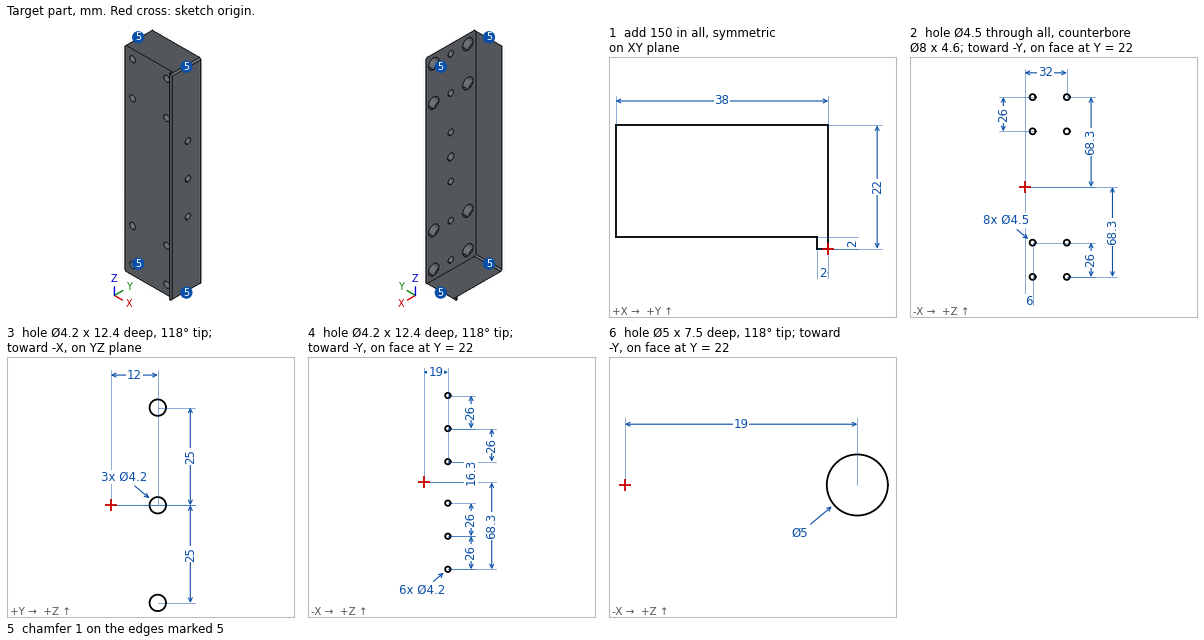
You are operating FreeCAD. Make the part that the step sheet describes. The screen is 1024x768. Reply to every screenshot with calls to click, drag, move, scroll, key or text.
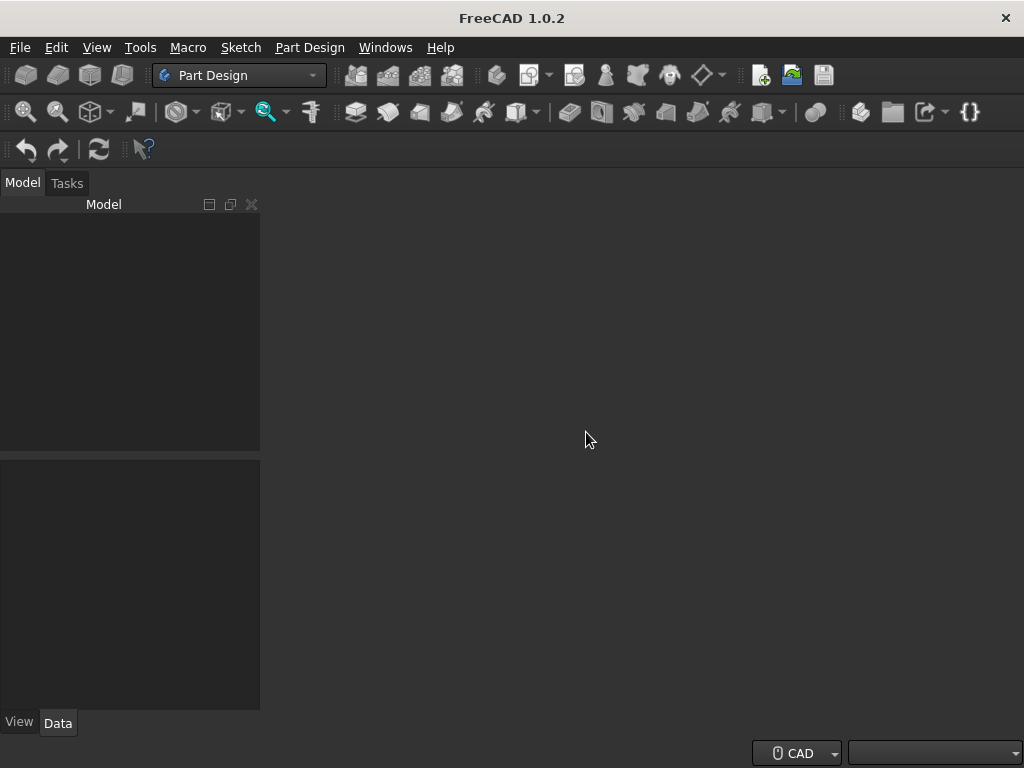
click(760, 76)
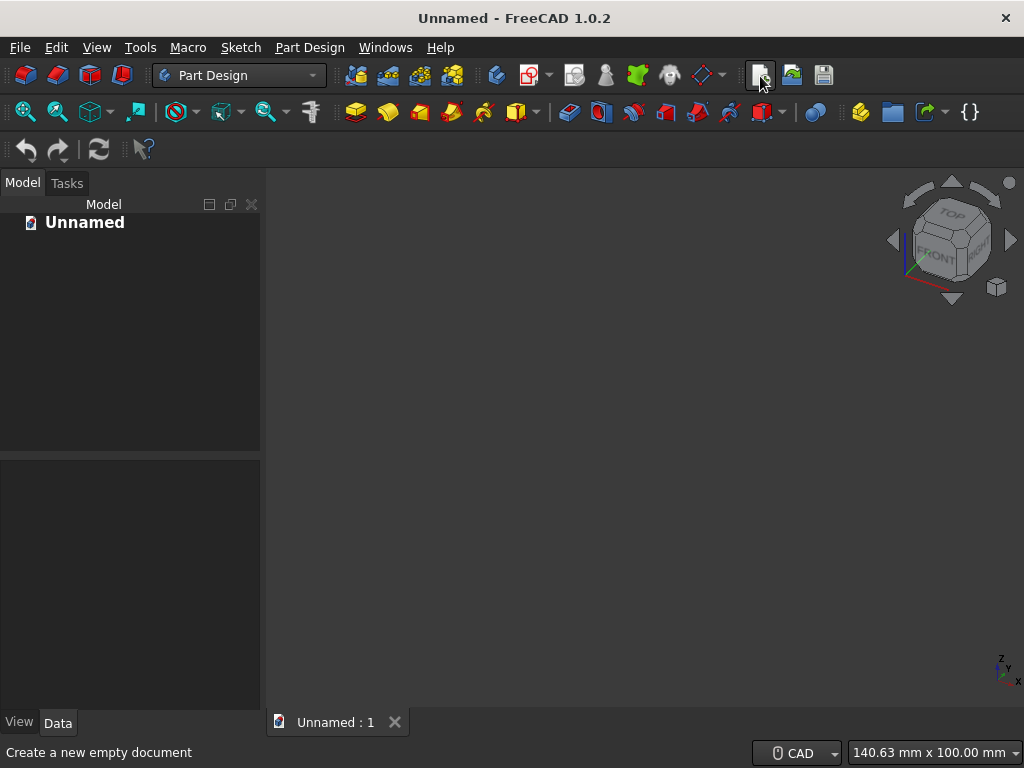
click(530, 76)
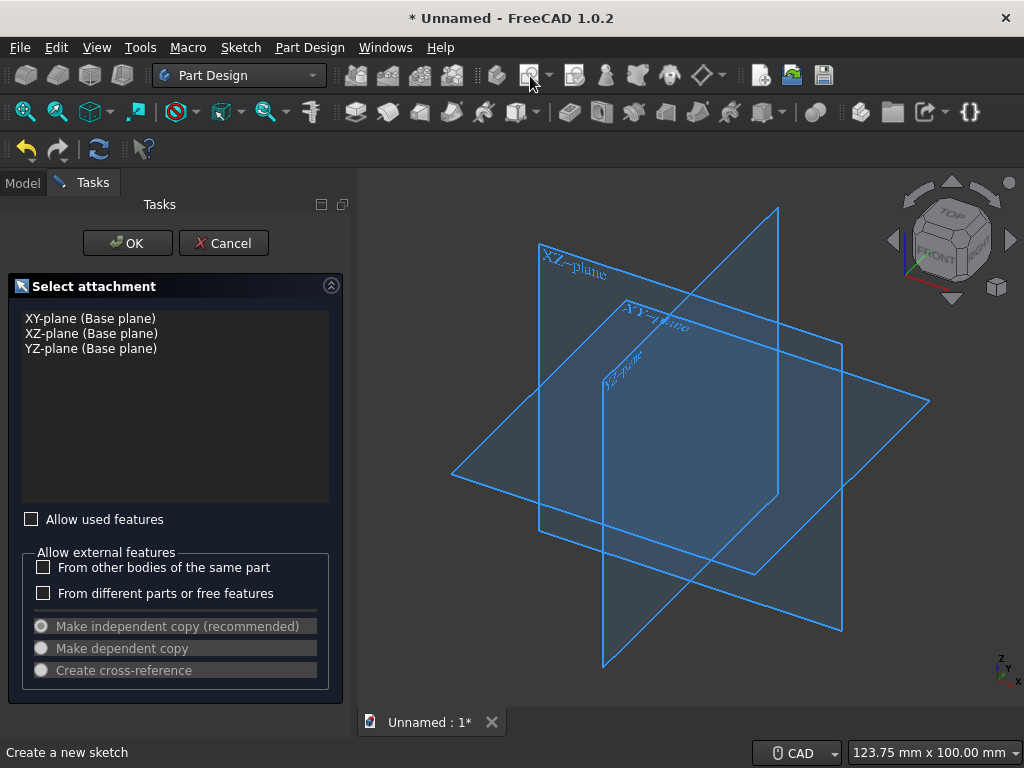
click(82, 318)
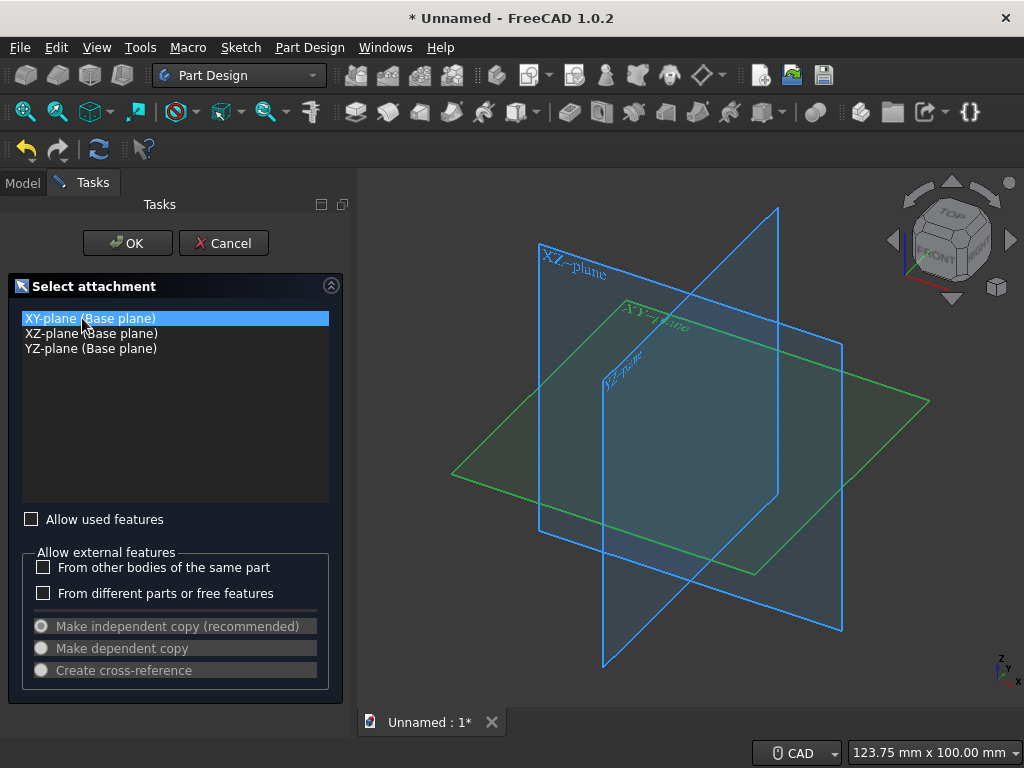
click(128, 243)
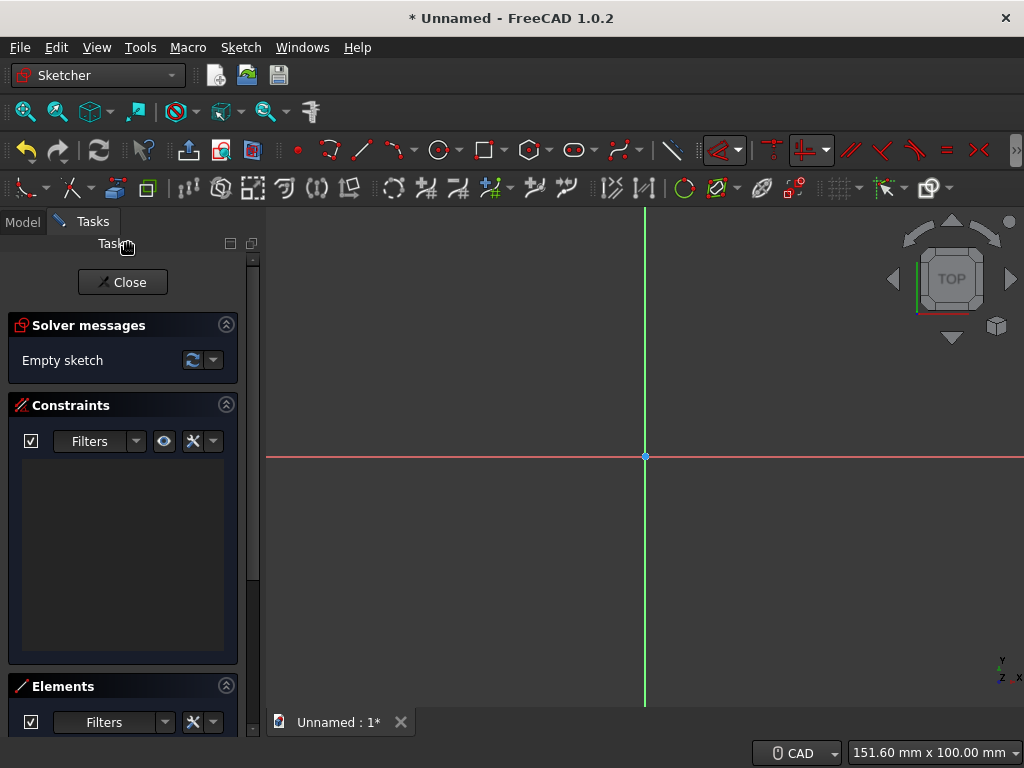
scroll(528, 357, up, 4)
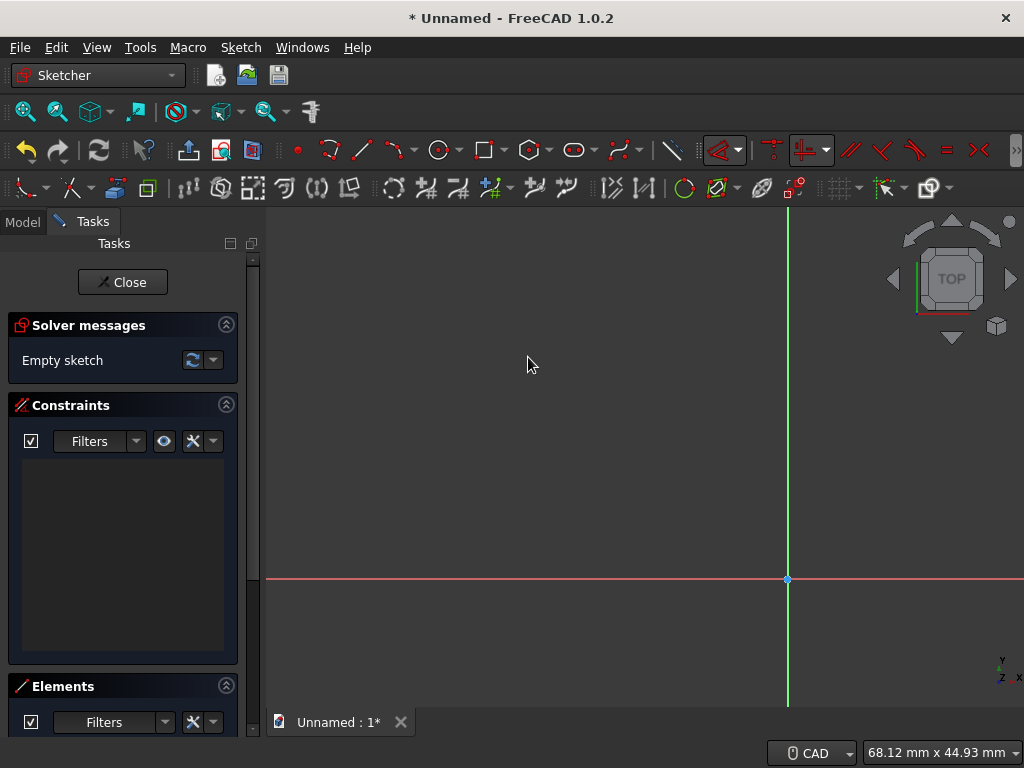
click(330, 150)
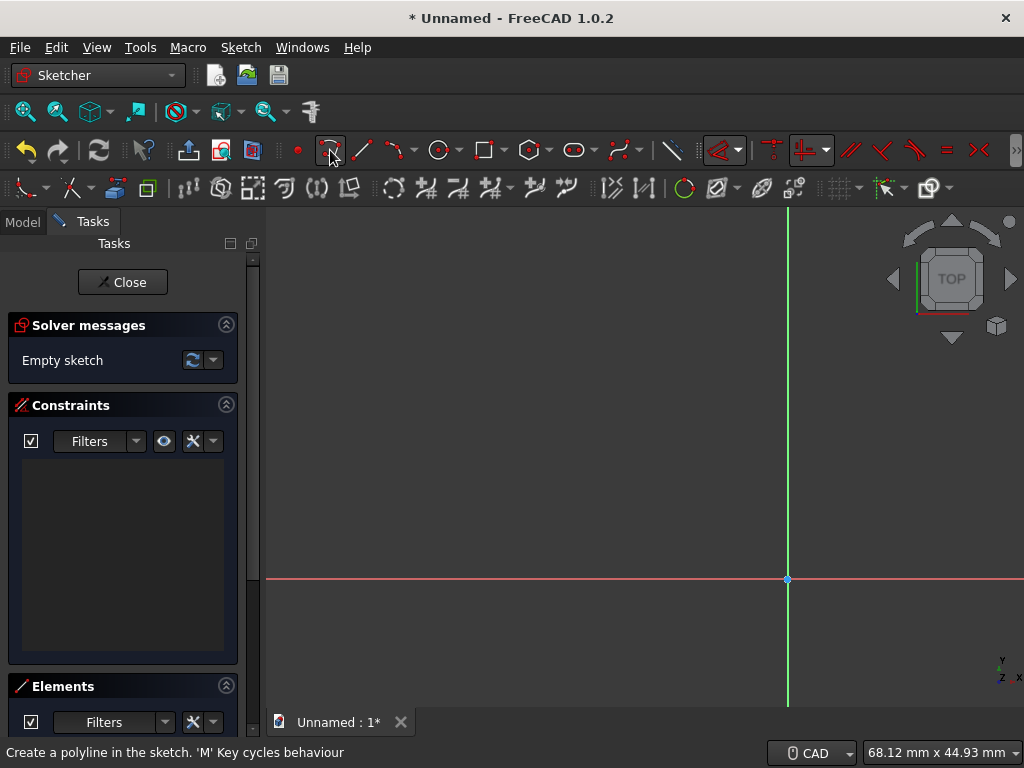
click(788, 579)
click(779, 334)
click(365, 334)
click(365, 557)
click(766, 557)
click(766, 570)
click(788, 579)
key(Escape)
key(Escape)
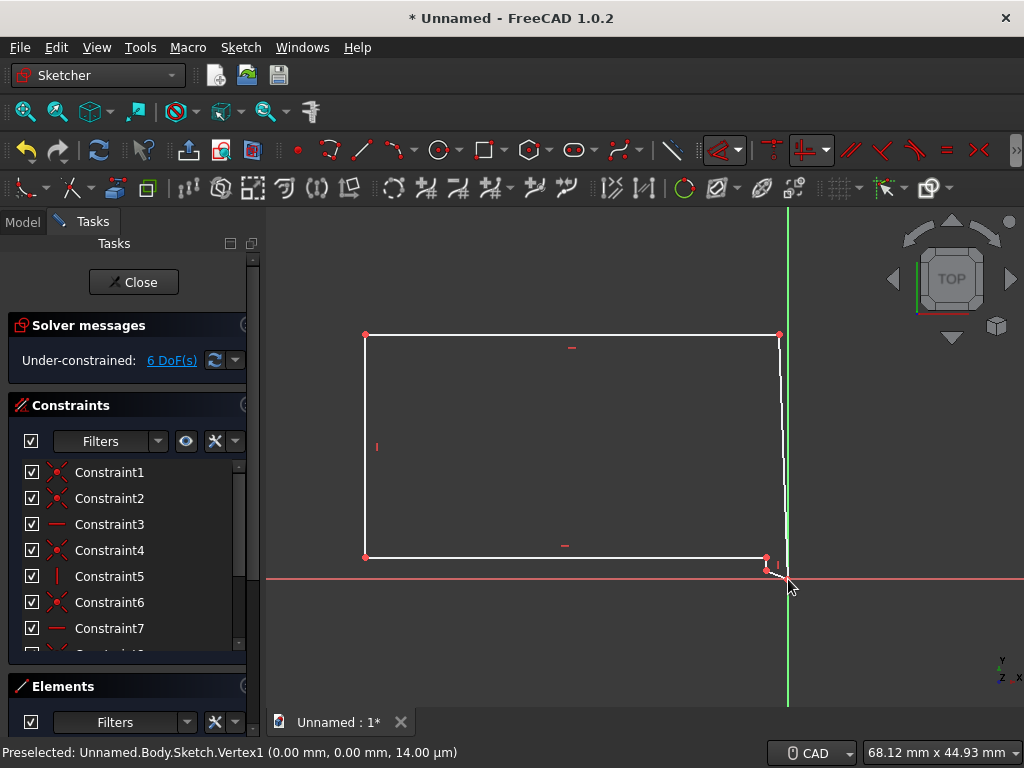
click(785, 506)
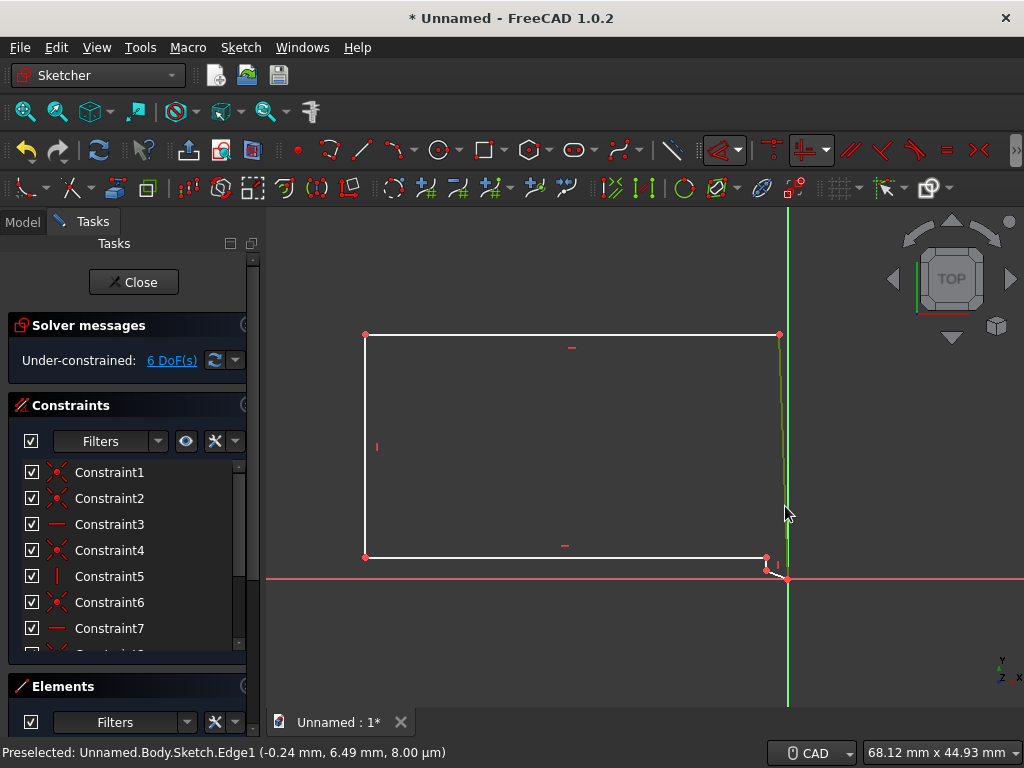
key(v)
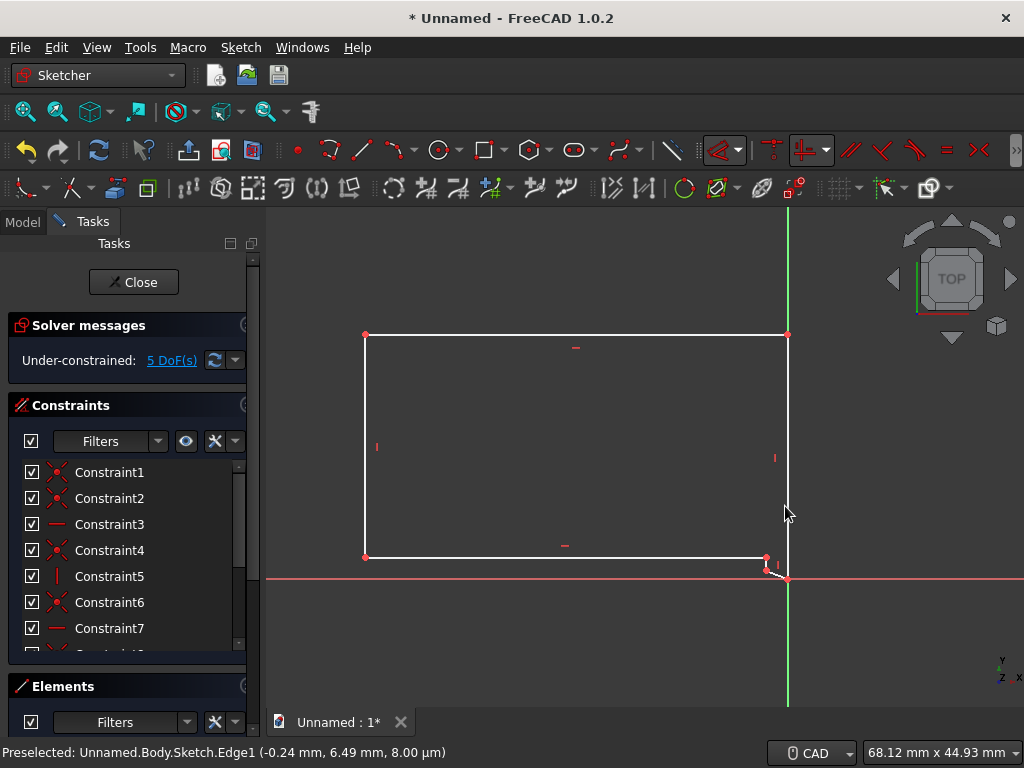
scroll(779, 576, up, 3)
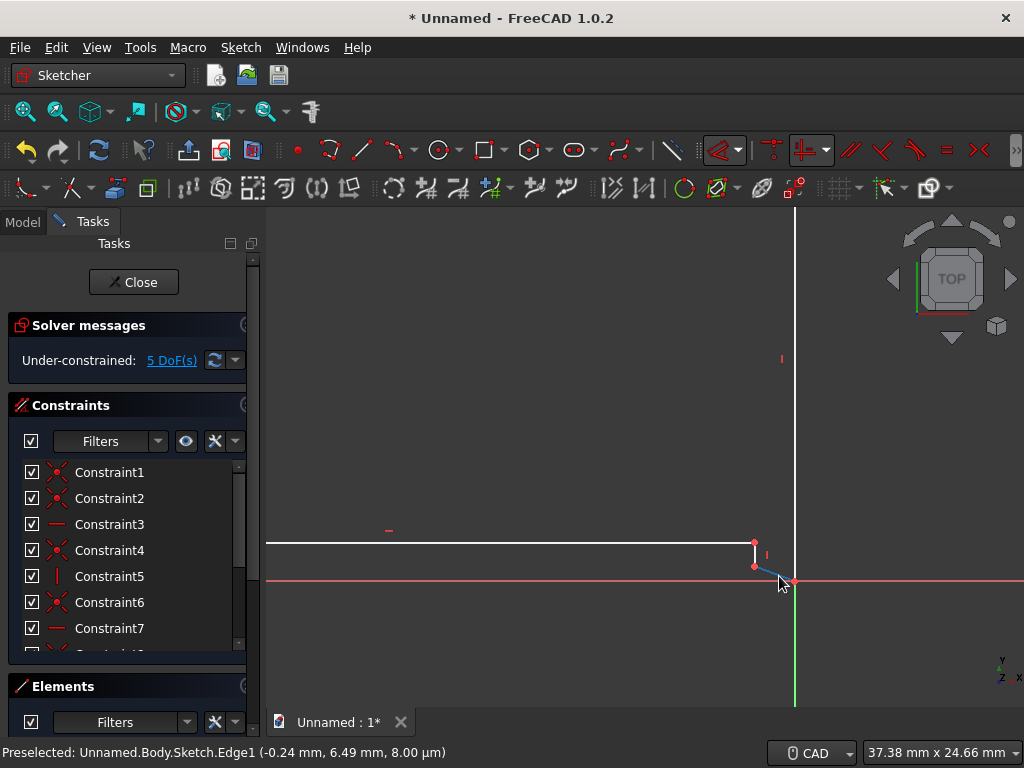
click(779, 575)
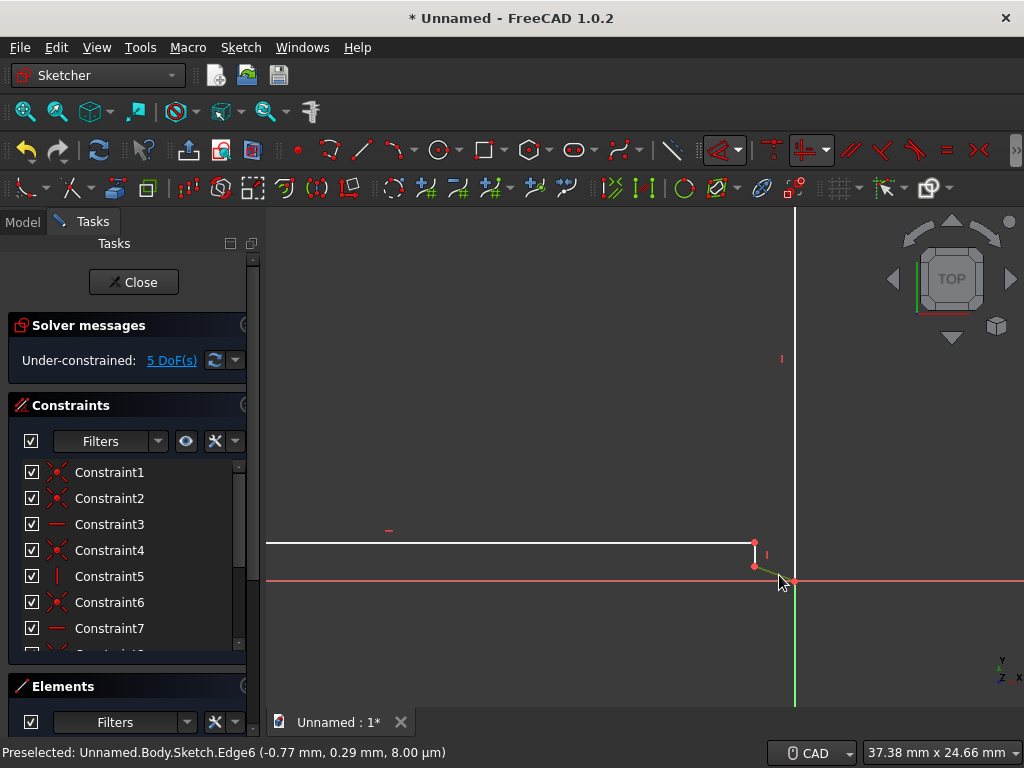
key(h)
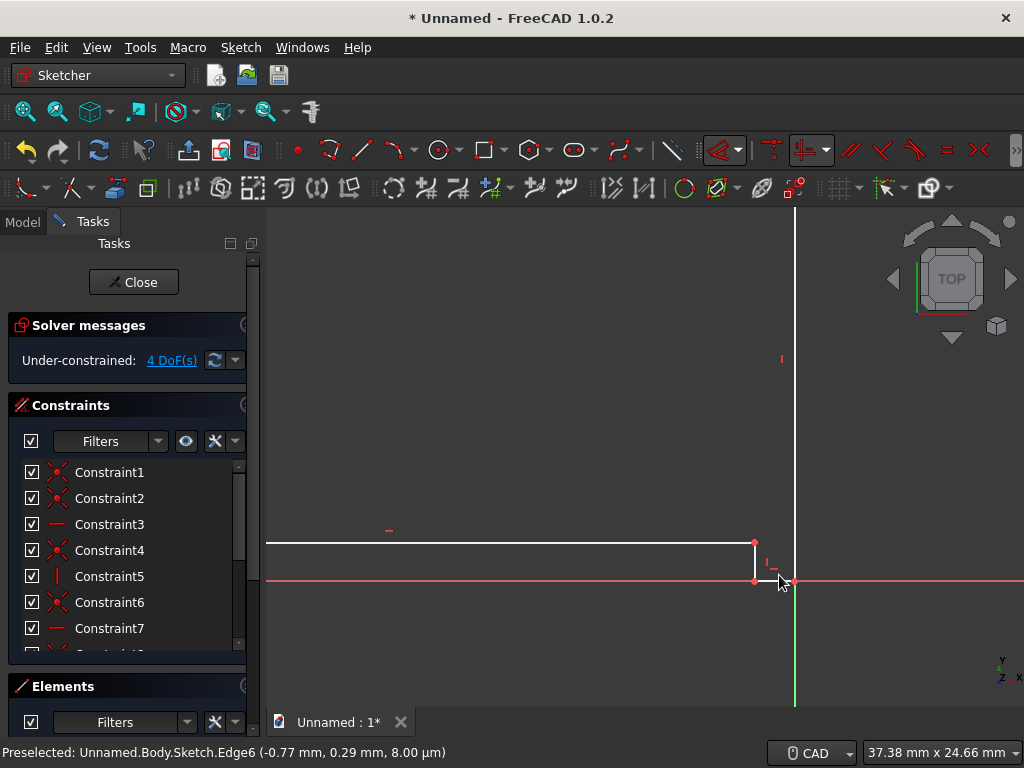
click(755, 554)